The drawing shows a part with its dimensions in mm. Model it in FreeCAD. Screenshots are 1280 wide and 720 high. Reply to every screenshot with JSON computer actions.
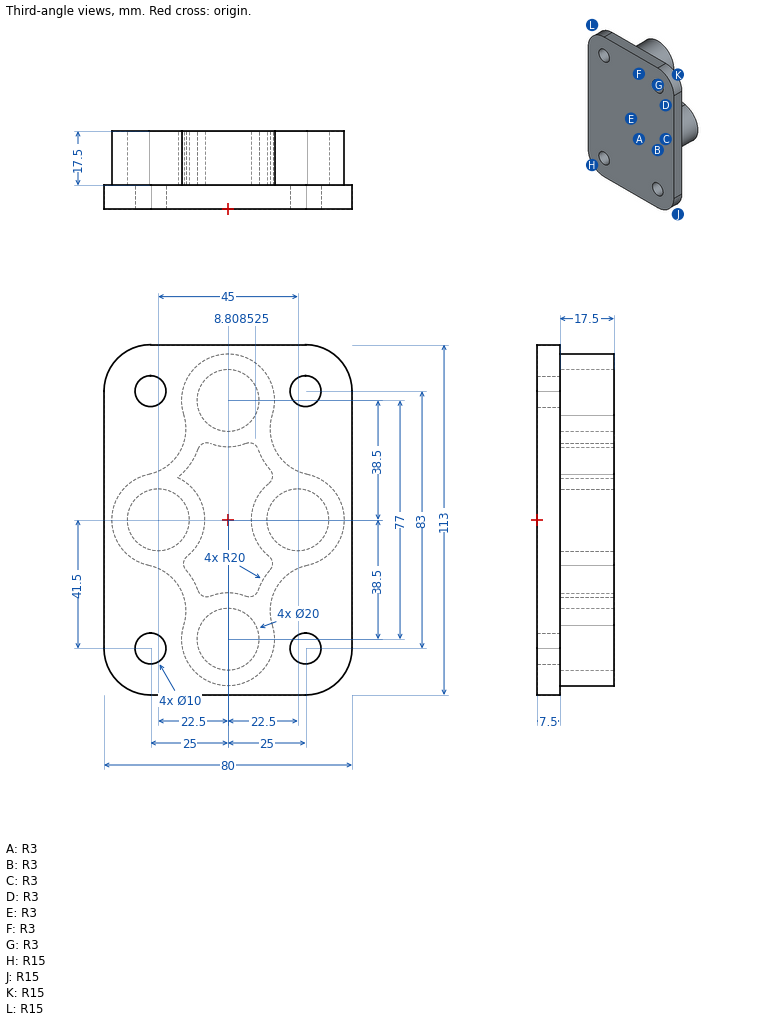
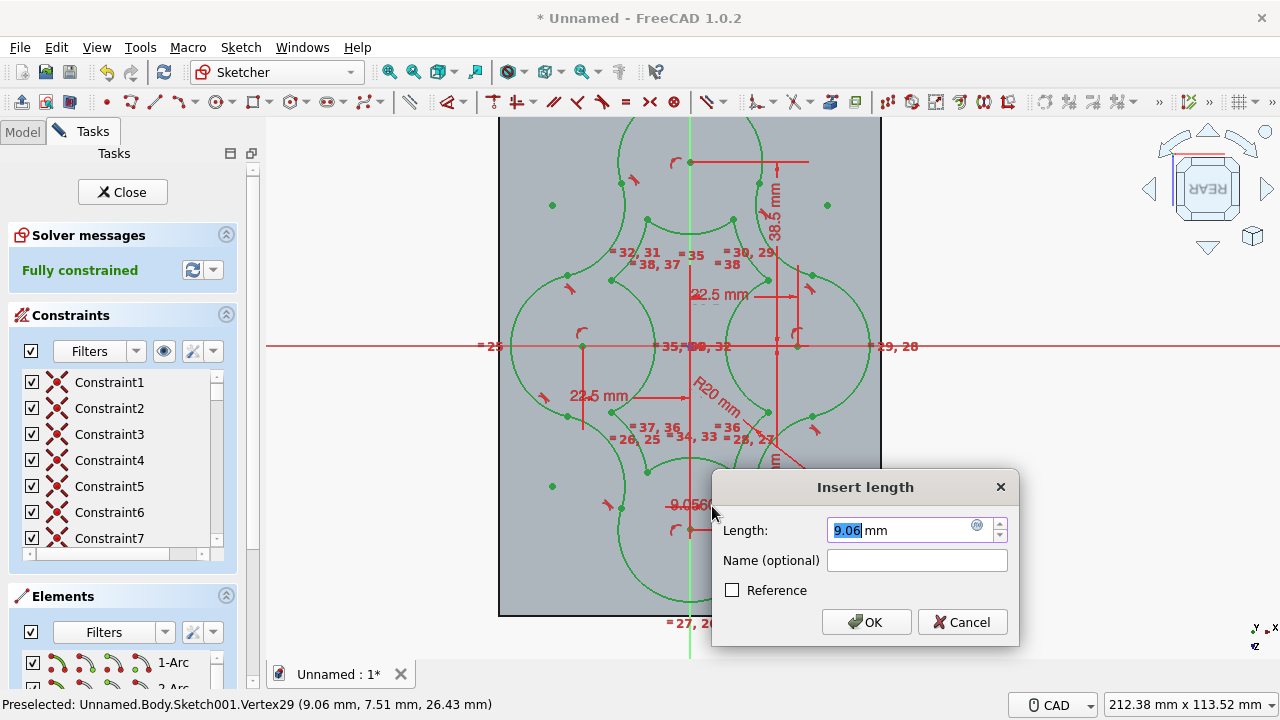
{"action": "type", "text": "8.808525"}
{"action": "key", "text": "Return"}
{"action": "key", "text": "Escape"}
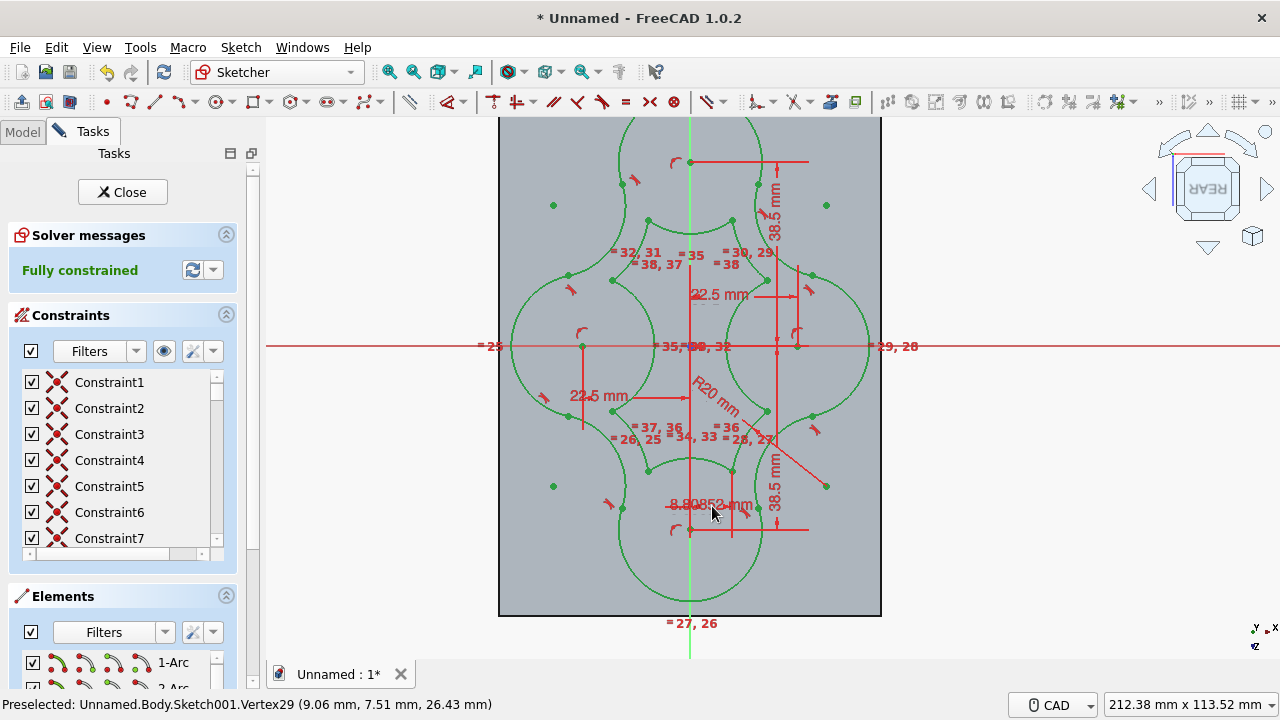
{"action": "left_click", "coordinate": [123, 192]}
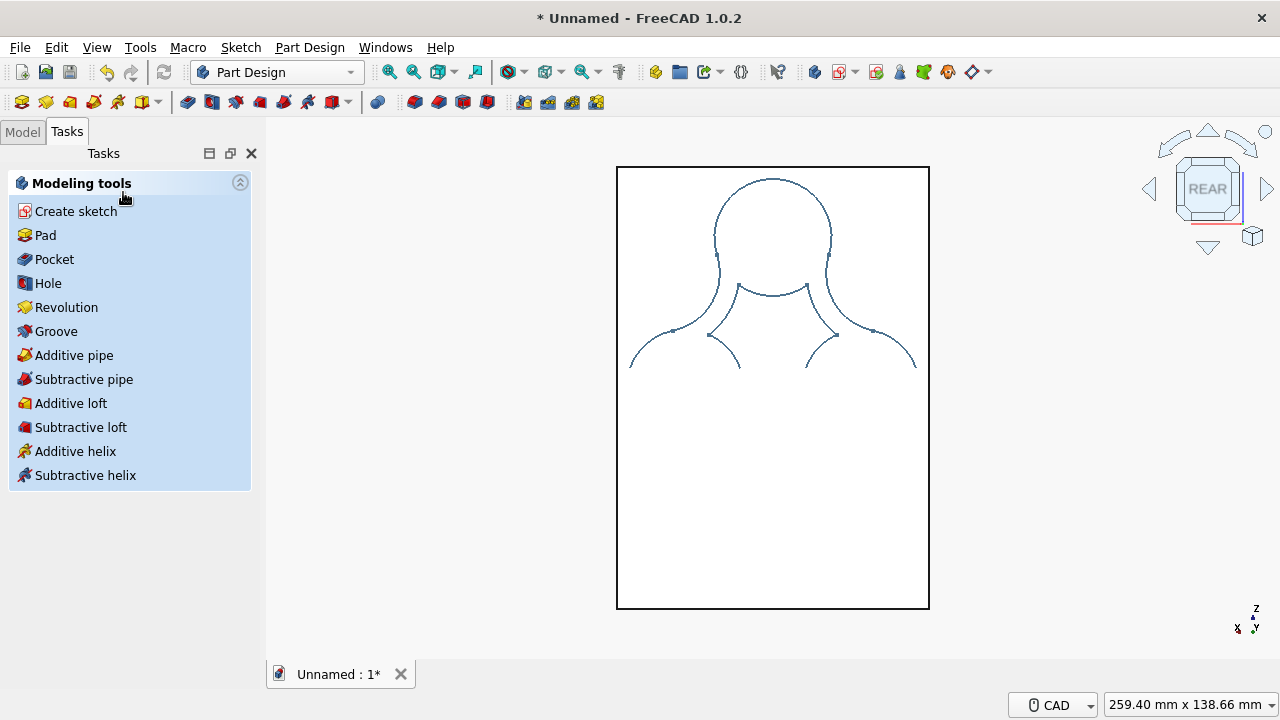
{"action": "left_click", "coordinate": [22, 102]}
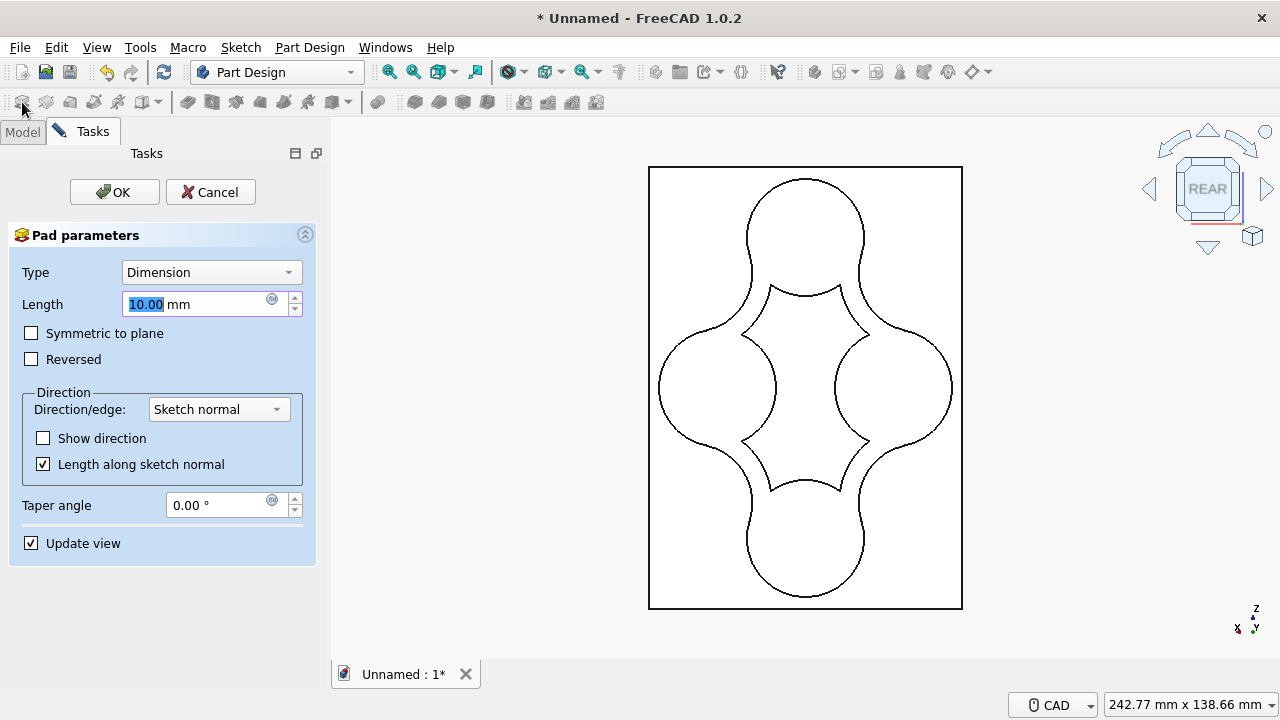
{"action": "type", "text": "17.5"}
{"action": "key", "text": "Tab"}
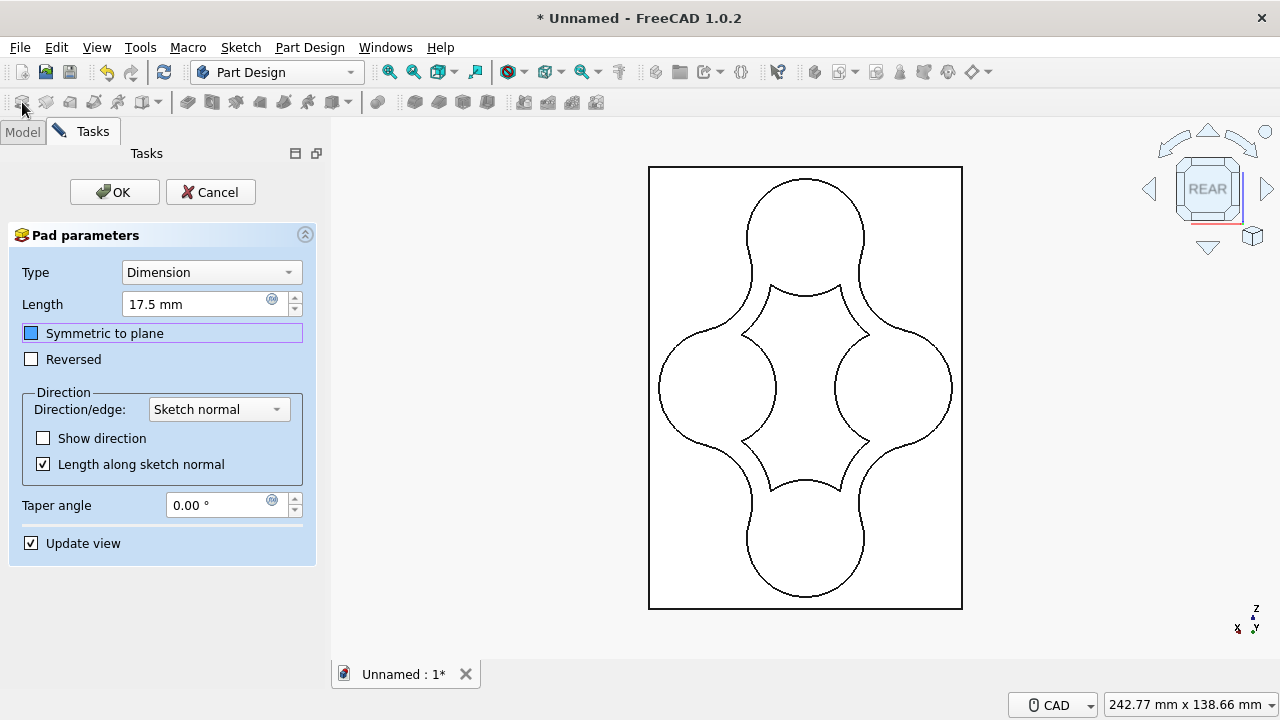
{"action": "left_click", "coordinate": [115, 192]}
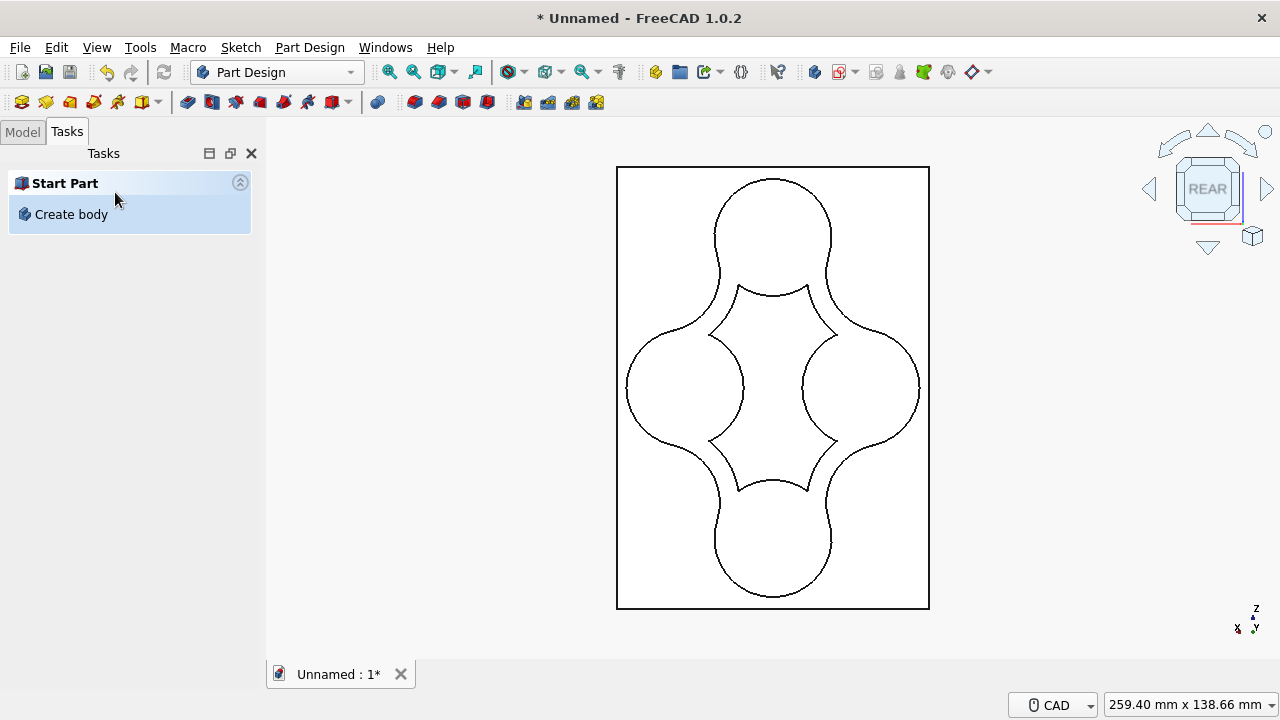
{"action": "key", "text": "0"}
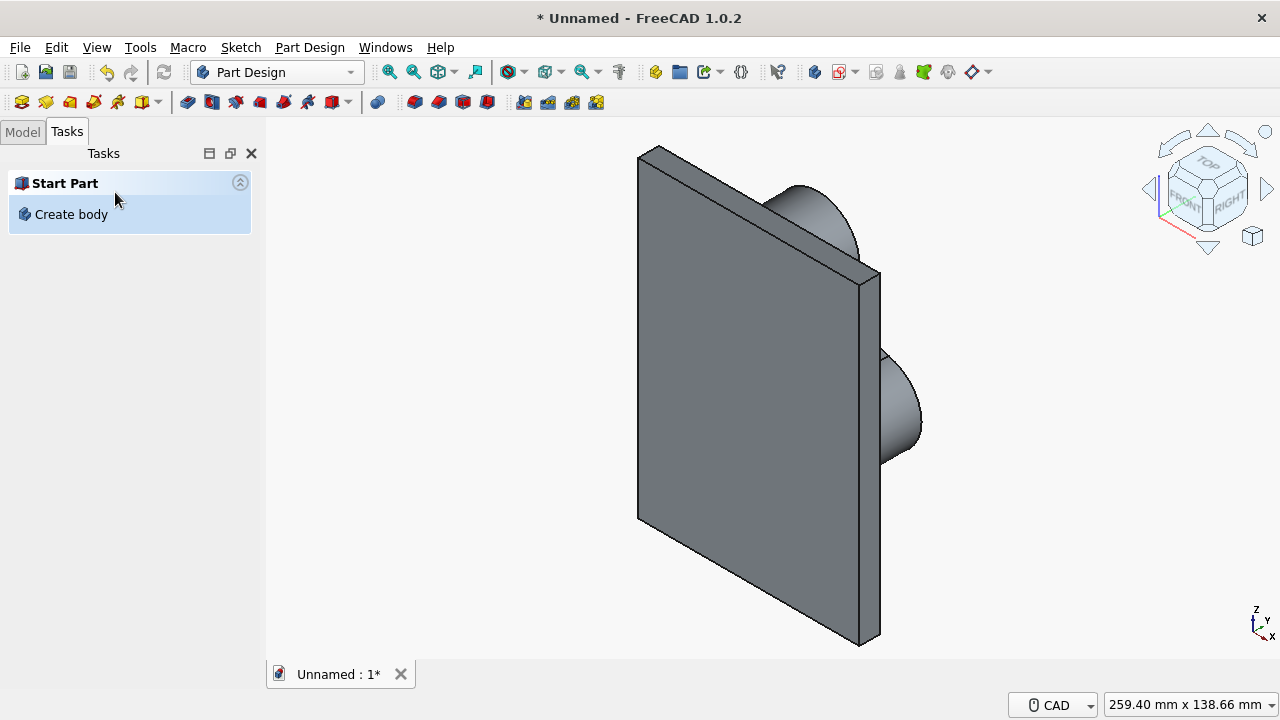
{"action": "key", "text": "2"}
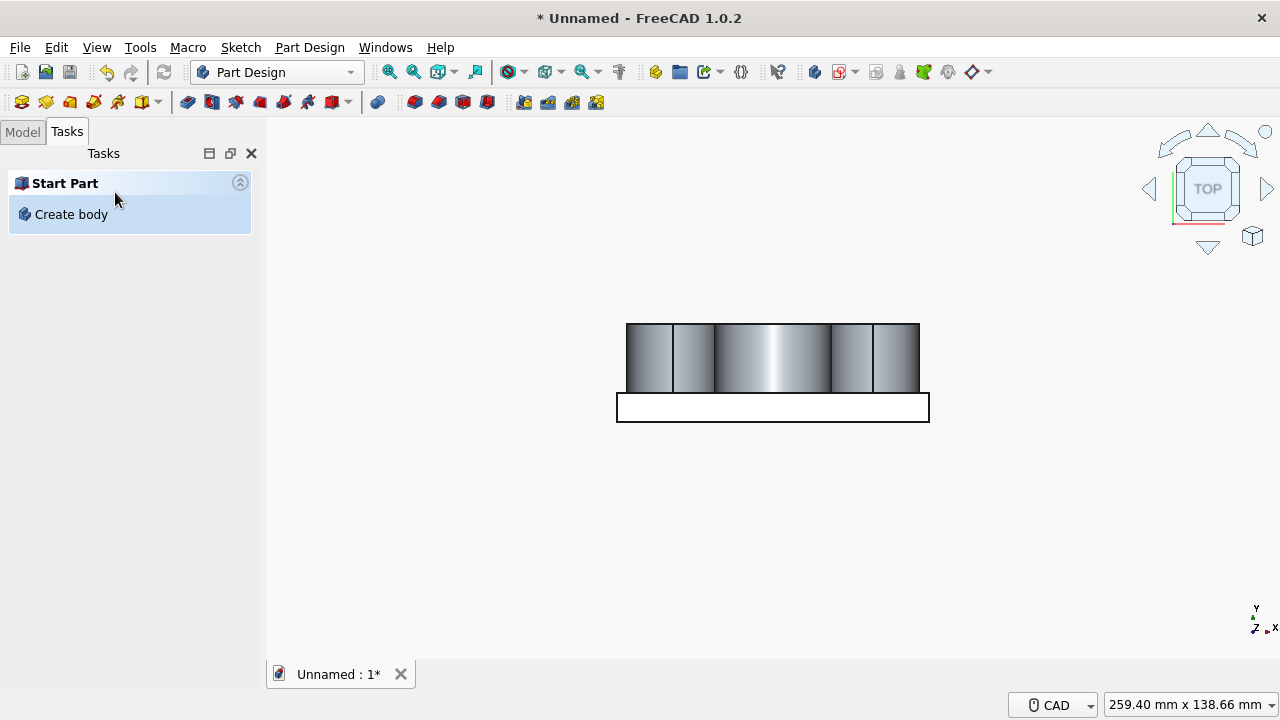
{"action": "key", "text": "v f"}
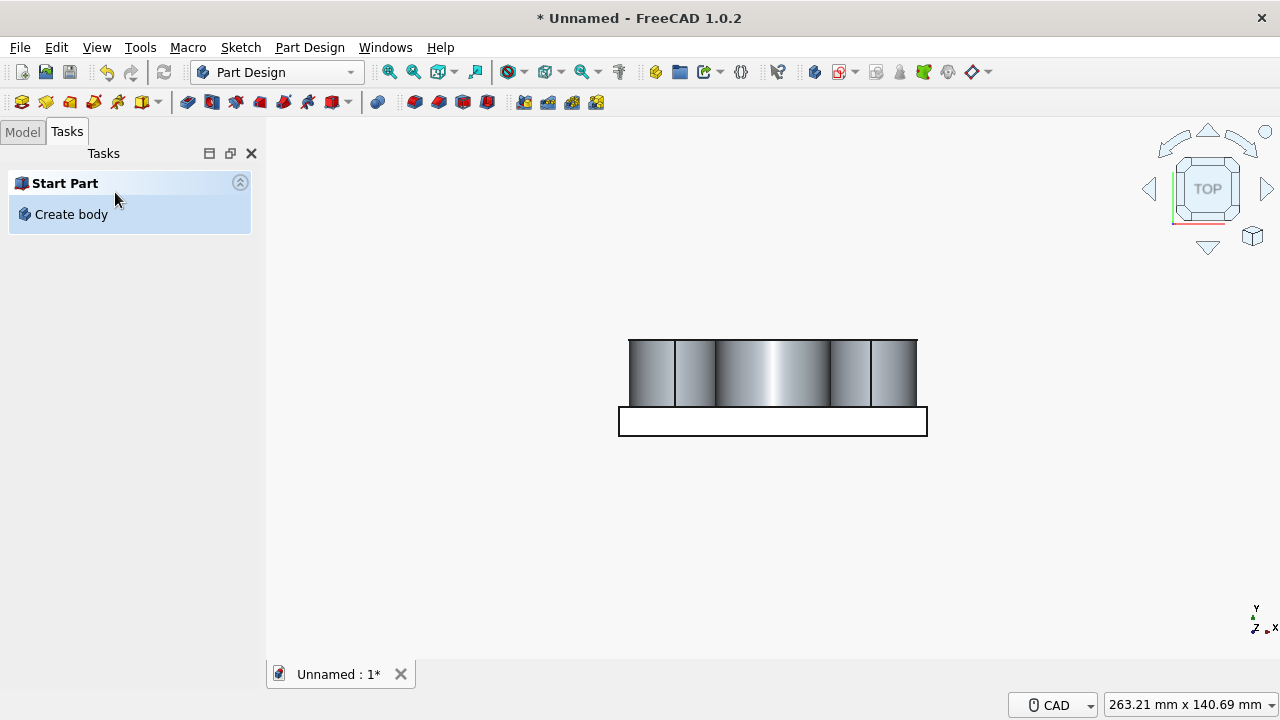
{"action": "key", "text": "1"}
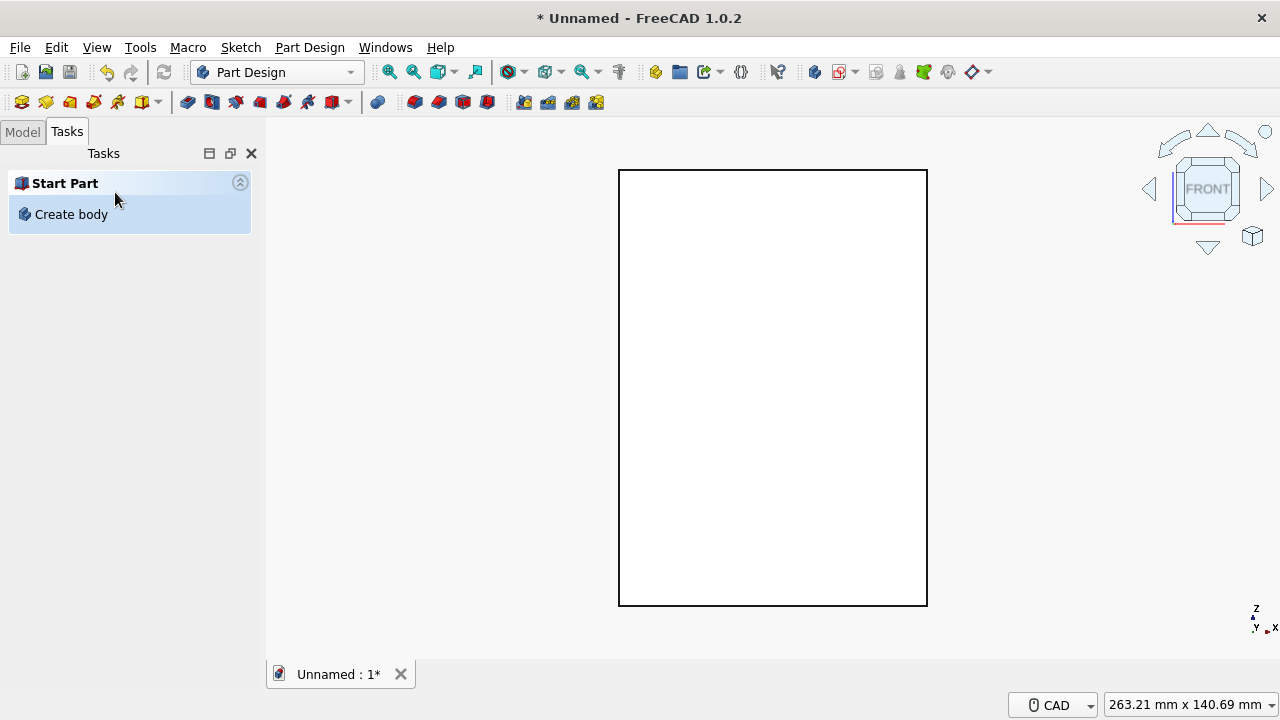
{"action": "key", "text": "3"}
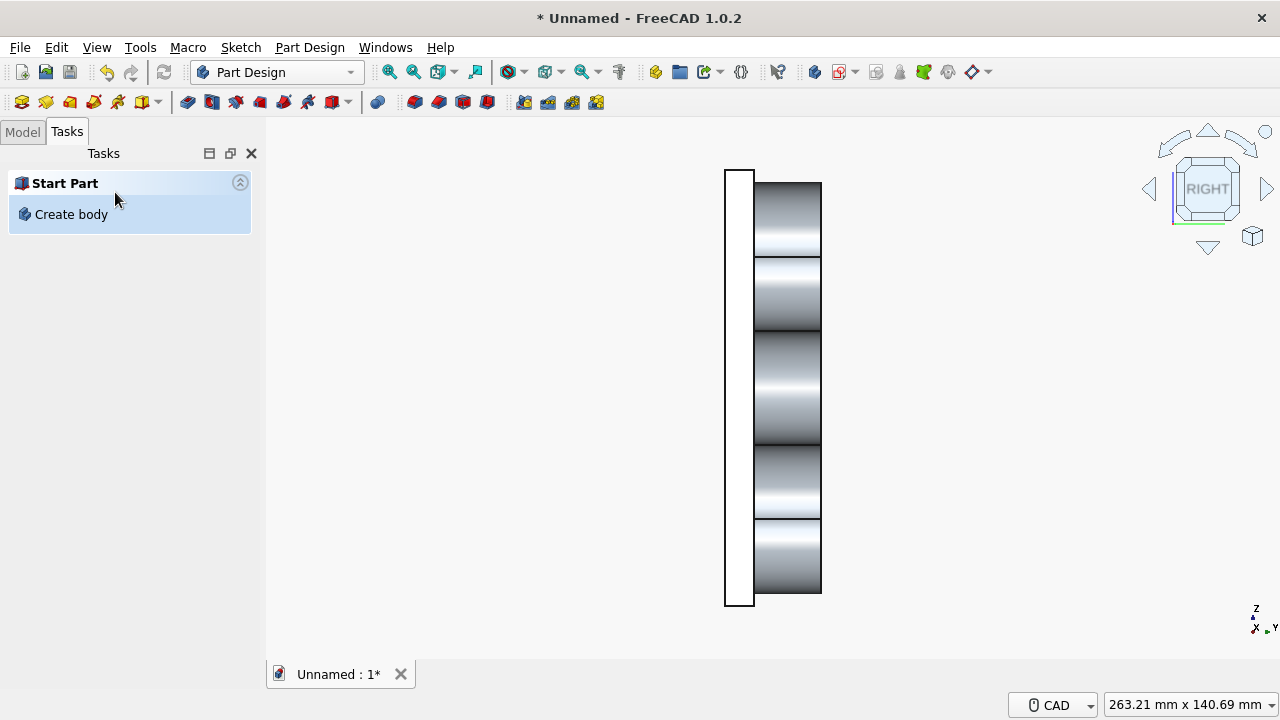
{"action": "key", "text": "5"}